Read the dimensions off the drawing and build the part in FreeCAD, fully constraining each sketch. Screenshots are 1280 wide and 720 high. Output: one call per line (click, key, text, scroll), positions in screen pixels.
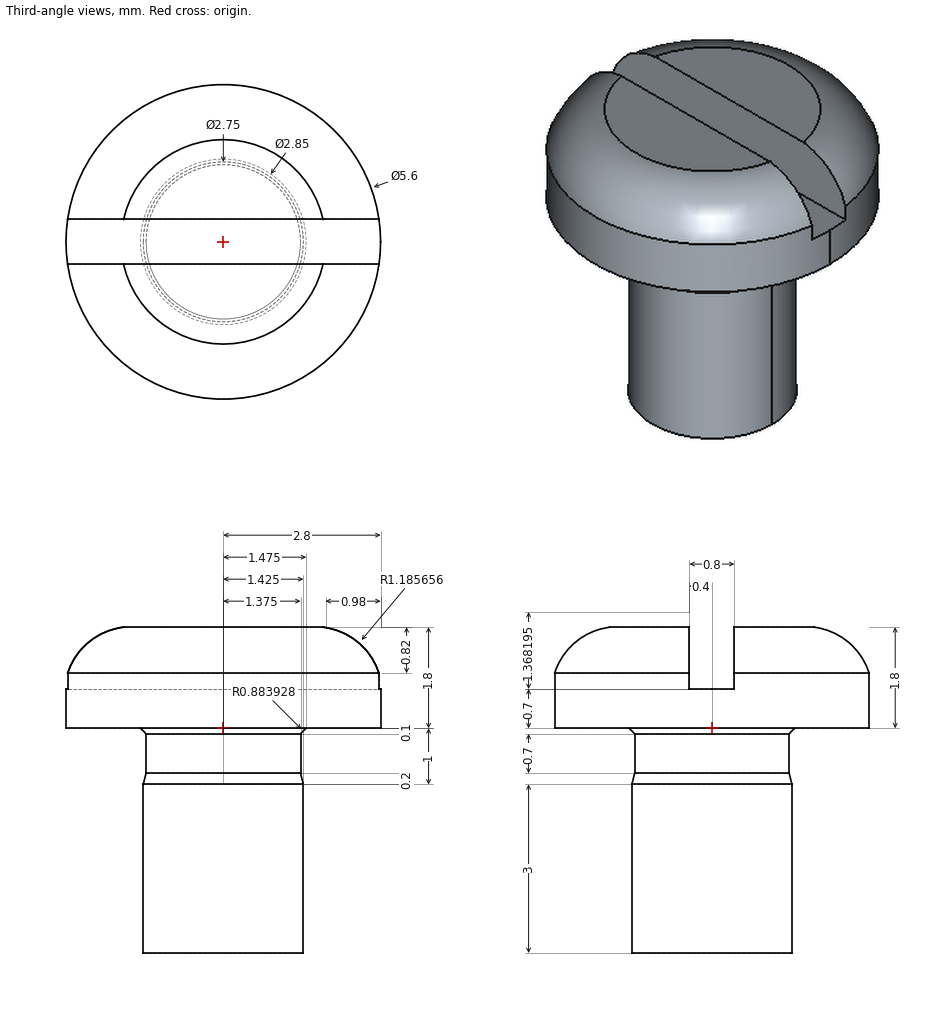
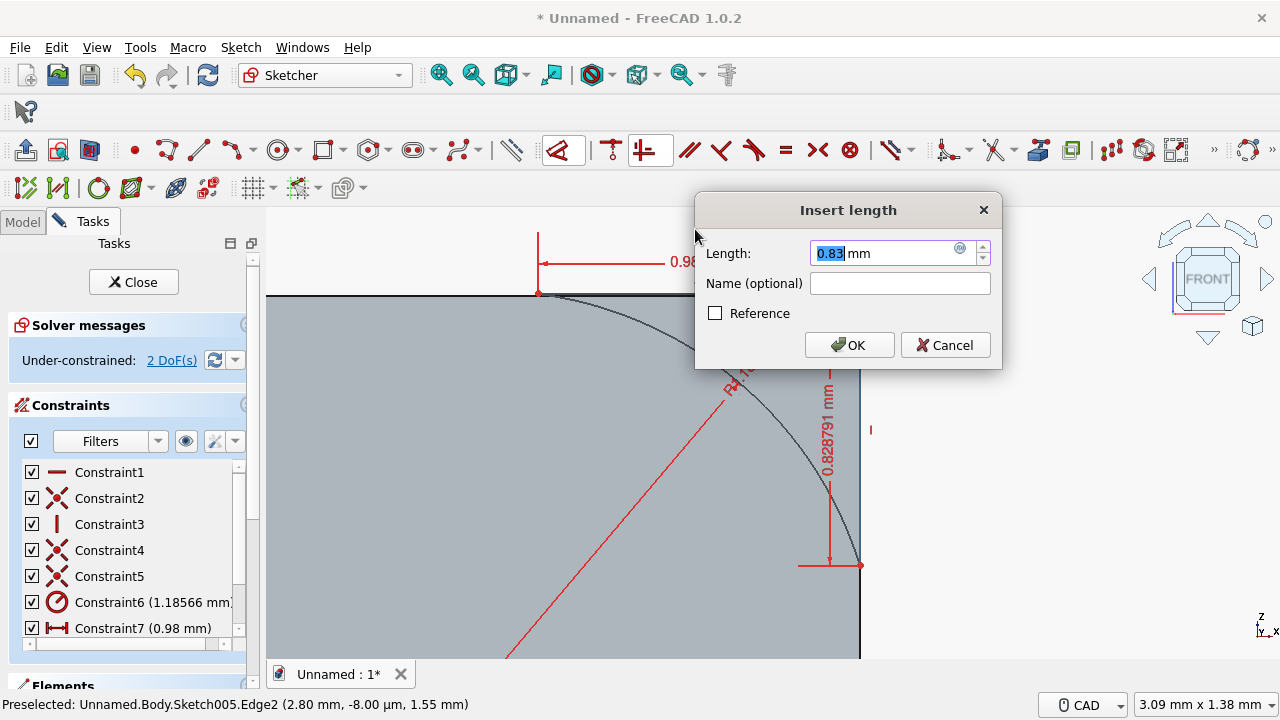
text(0.82)
key(Return)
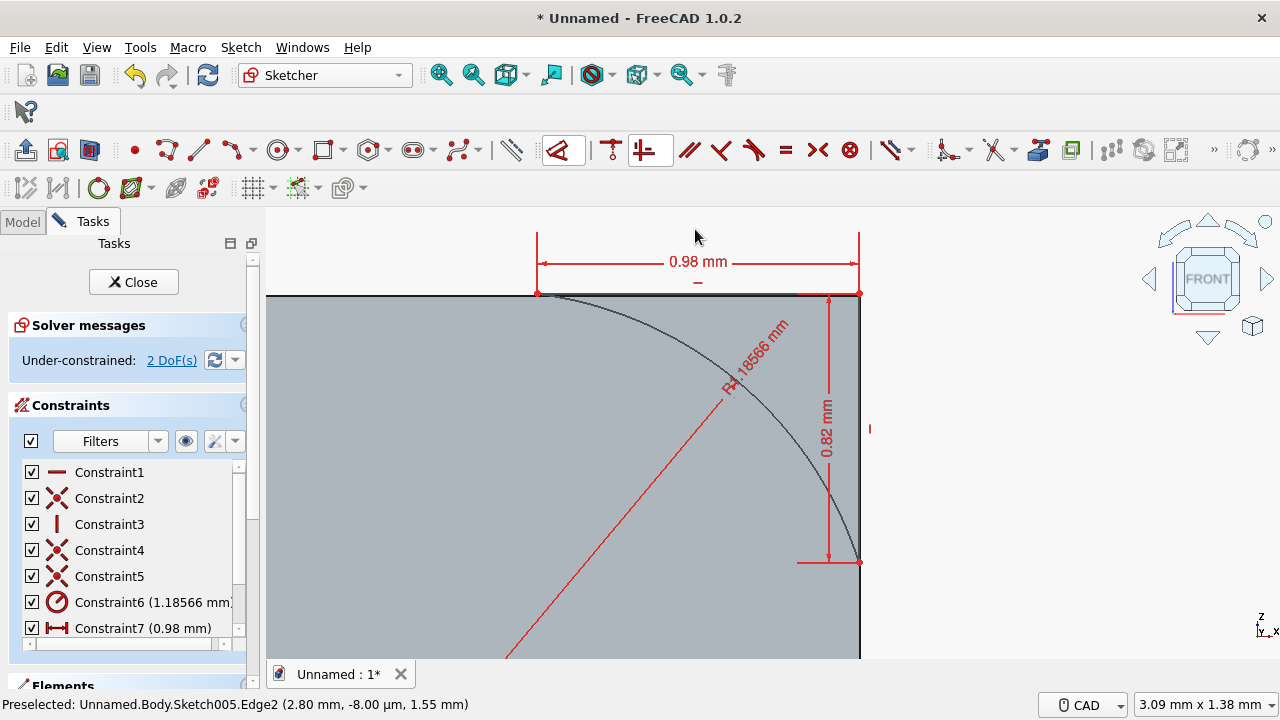
click(537, 294)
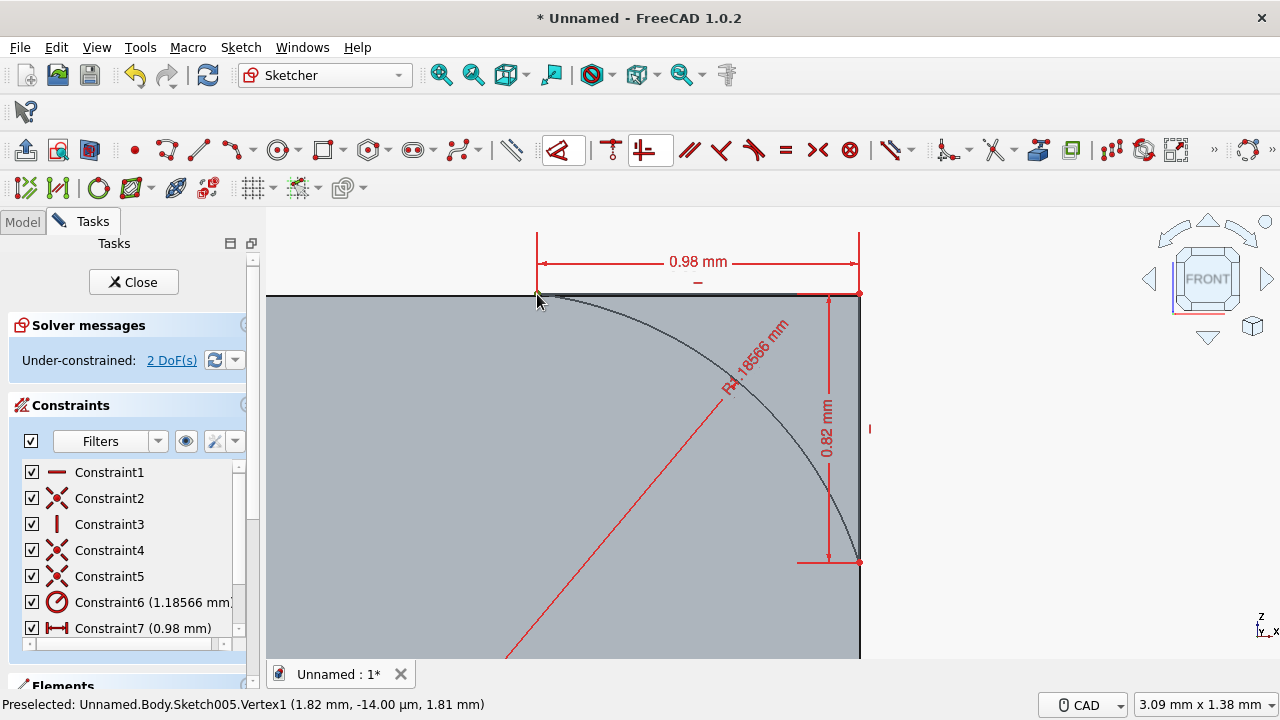
click(580, 150)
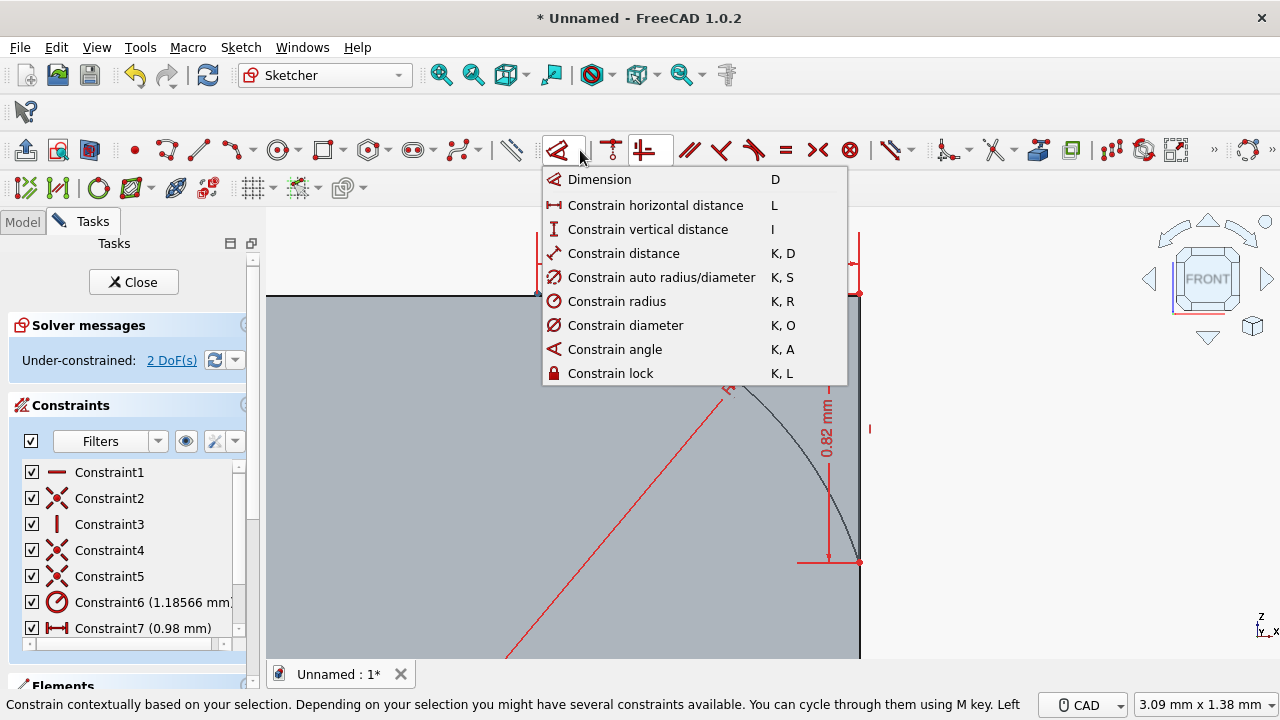
click(695, 229)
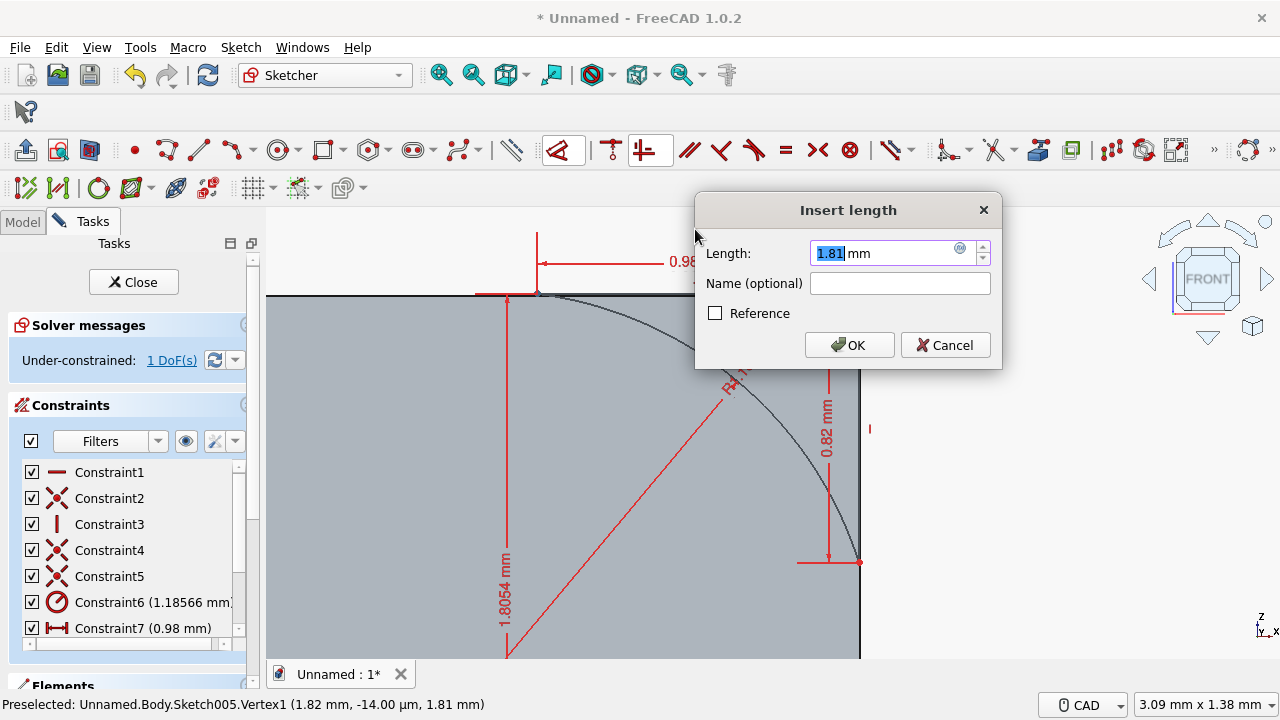
text(1.8)
key(Return)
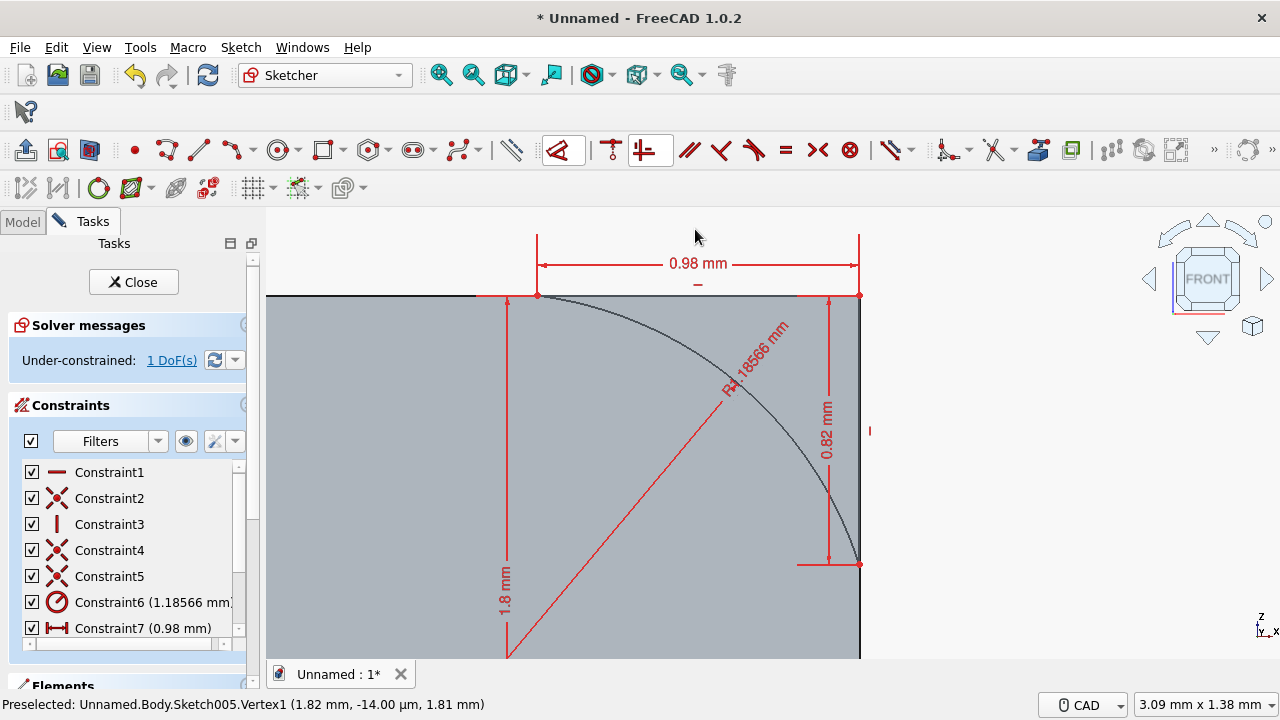
click(859, 296)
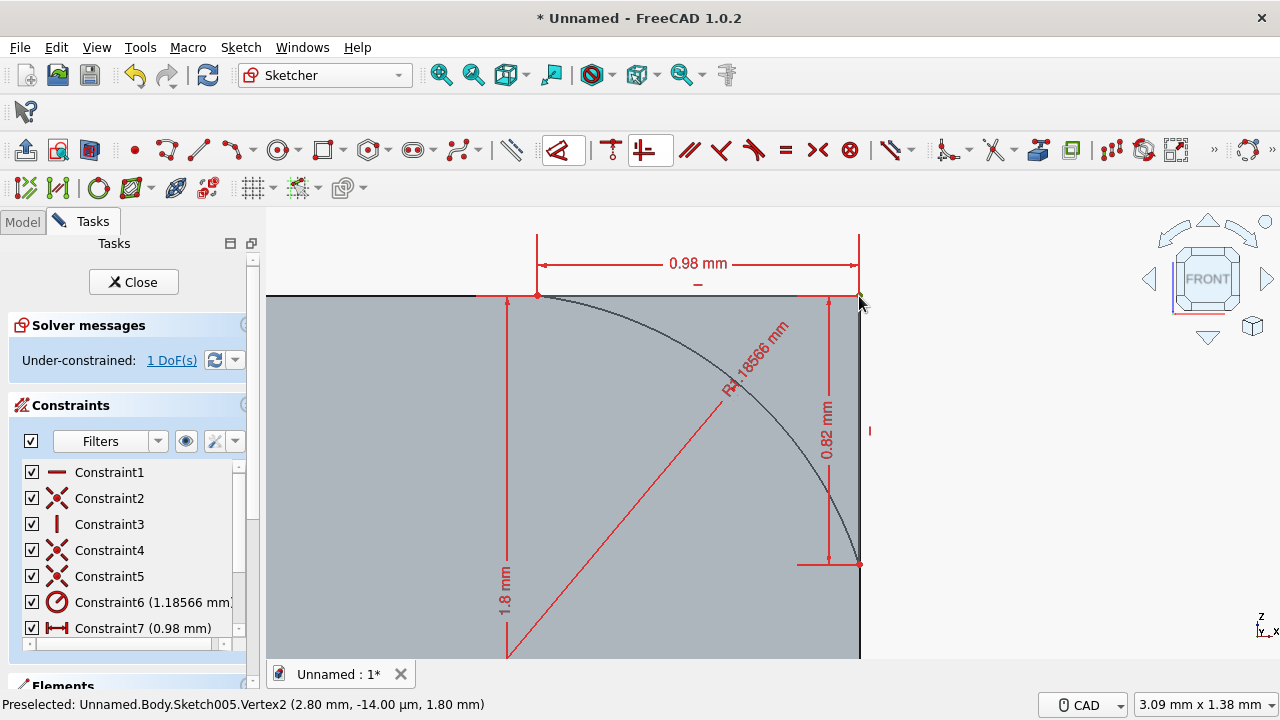
key(l)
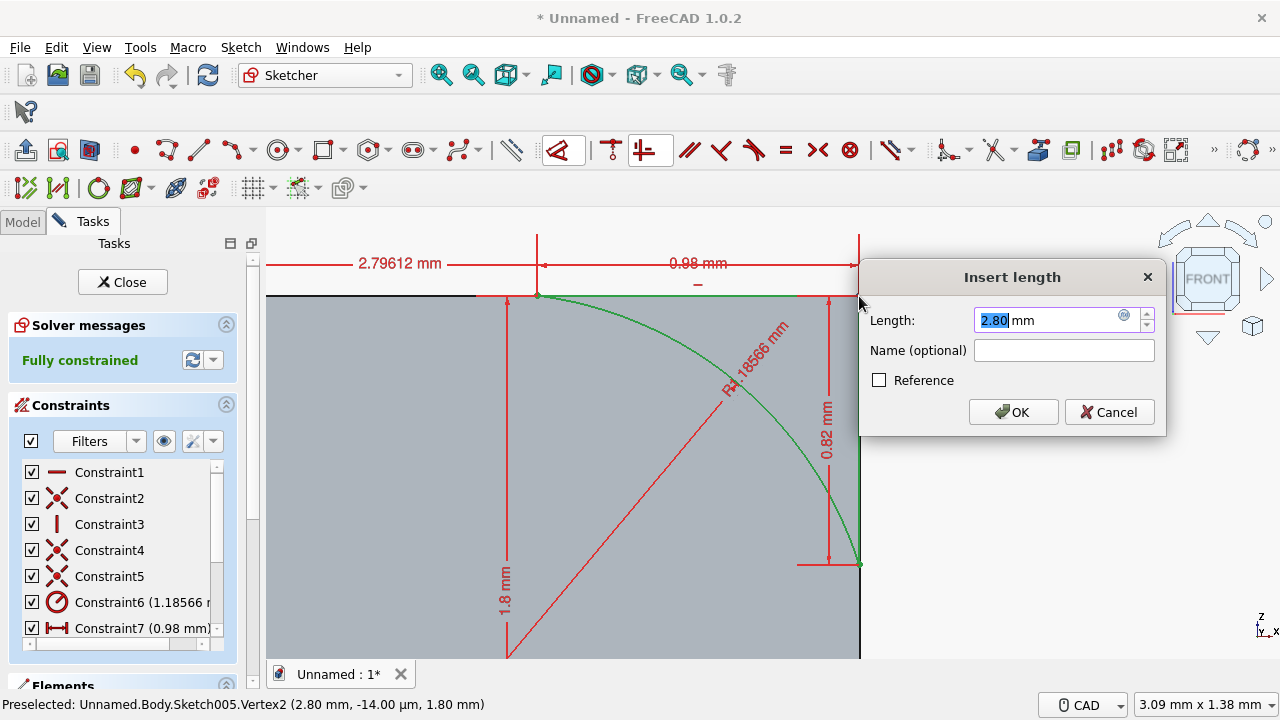
text(2.8)
key(Return)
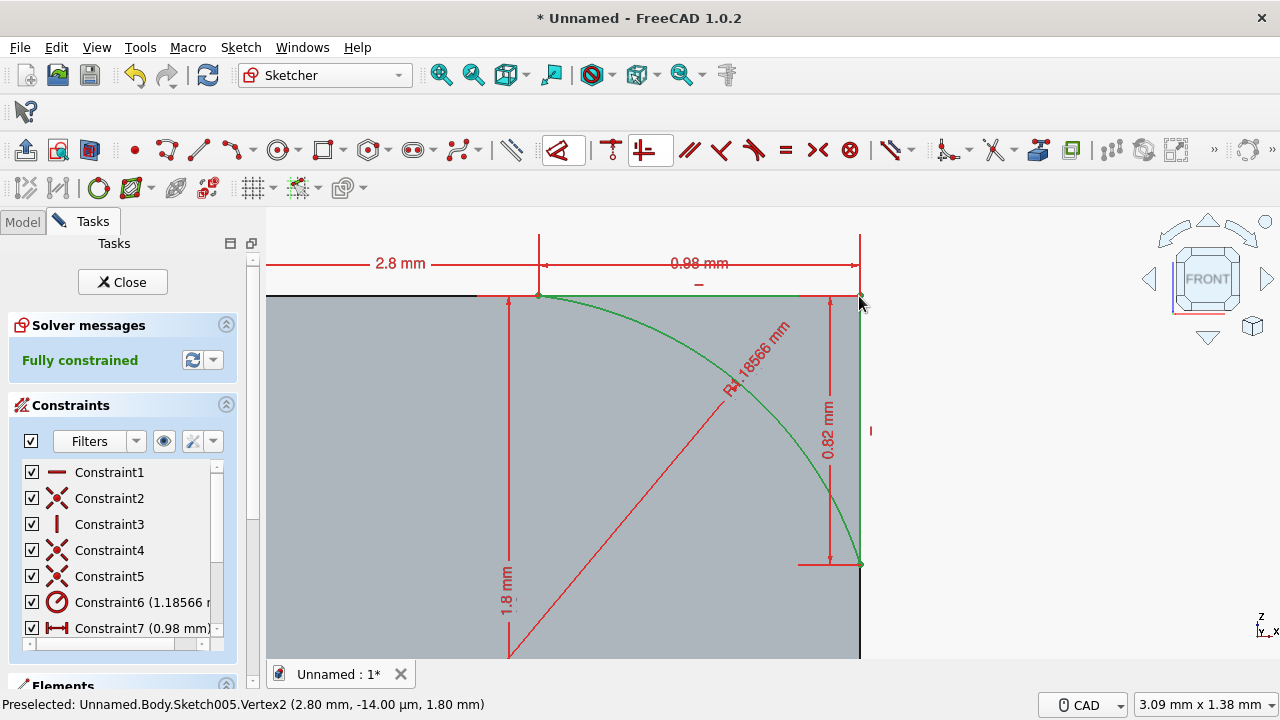
click(123, 282)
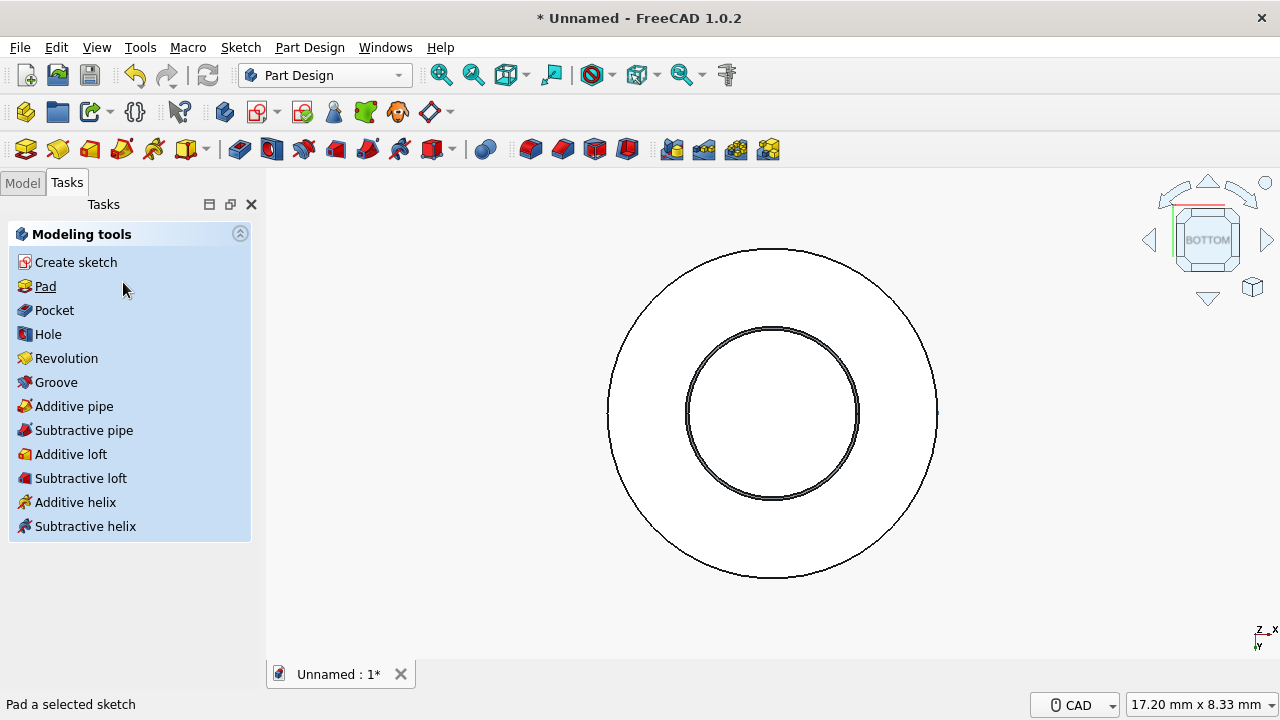
click(304, 150)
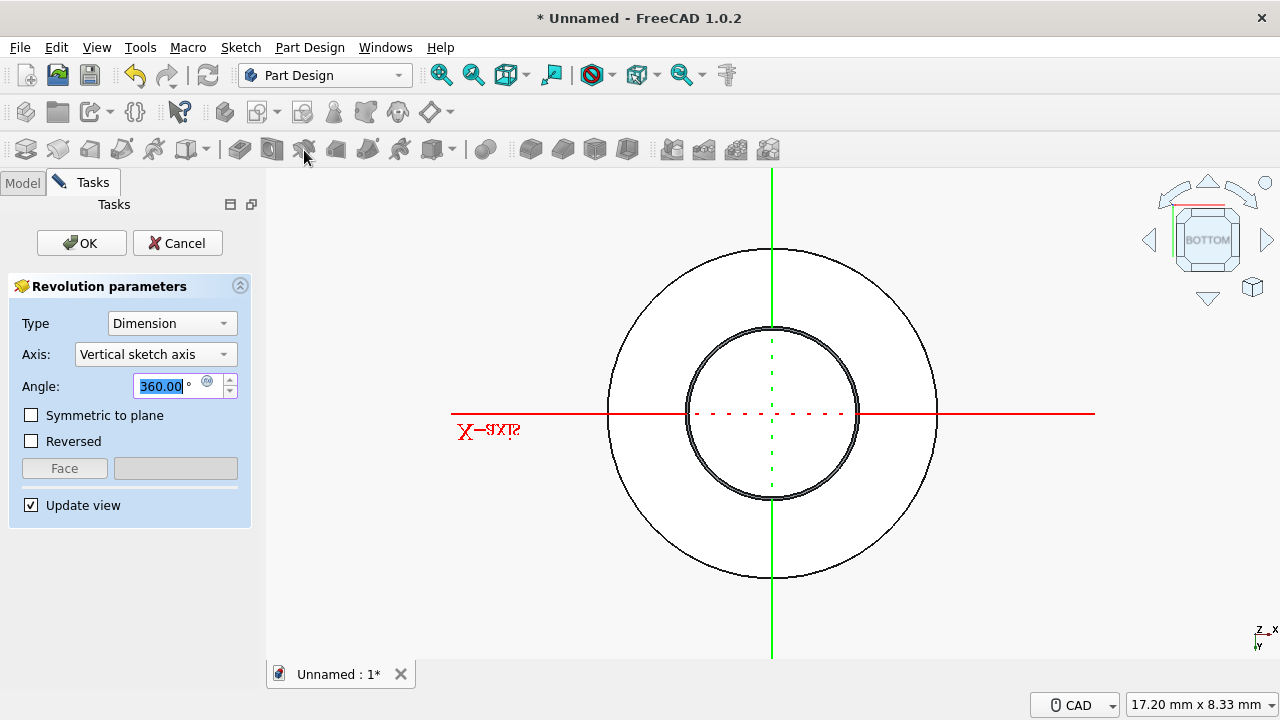
click(82, 243)